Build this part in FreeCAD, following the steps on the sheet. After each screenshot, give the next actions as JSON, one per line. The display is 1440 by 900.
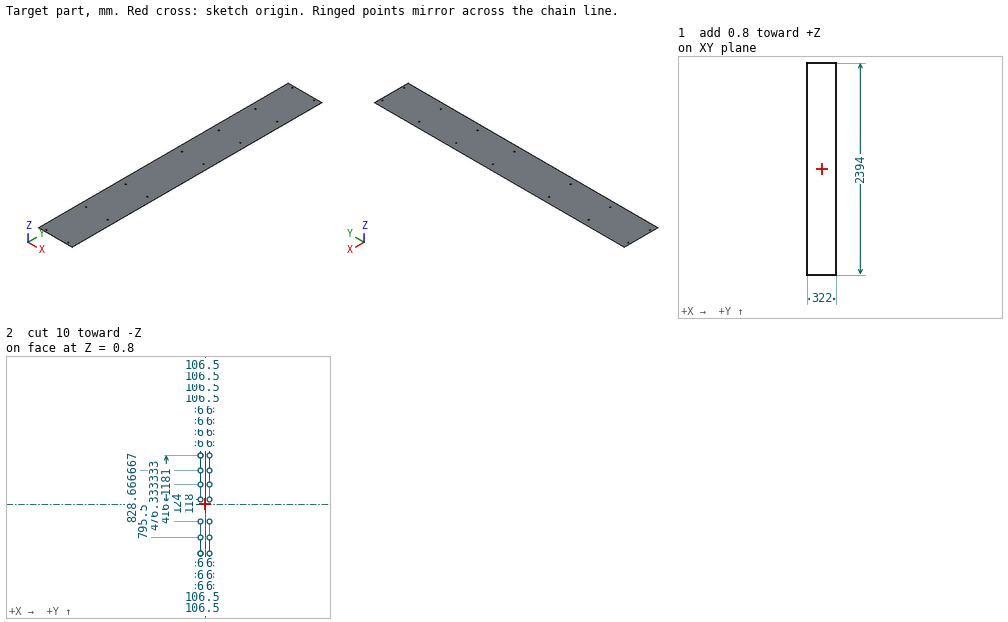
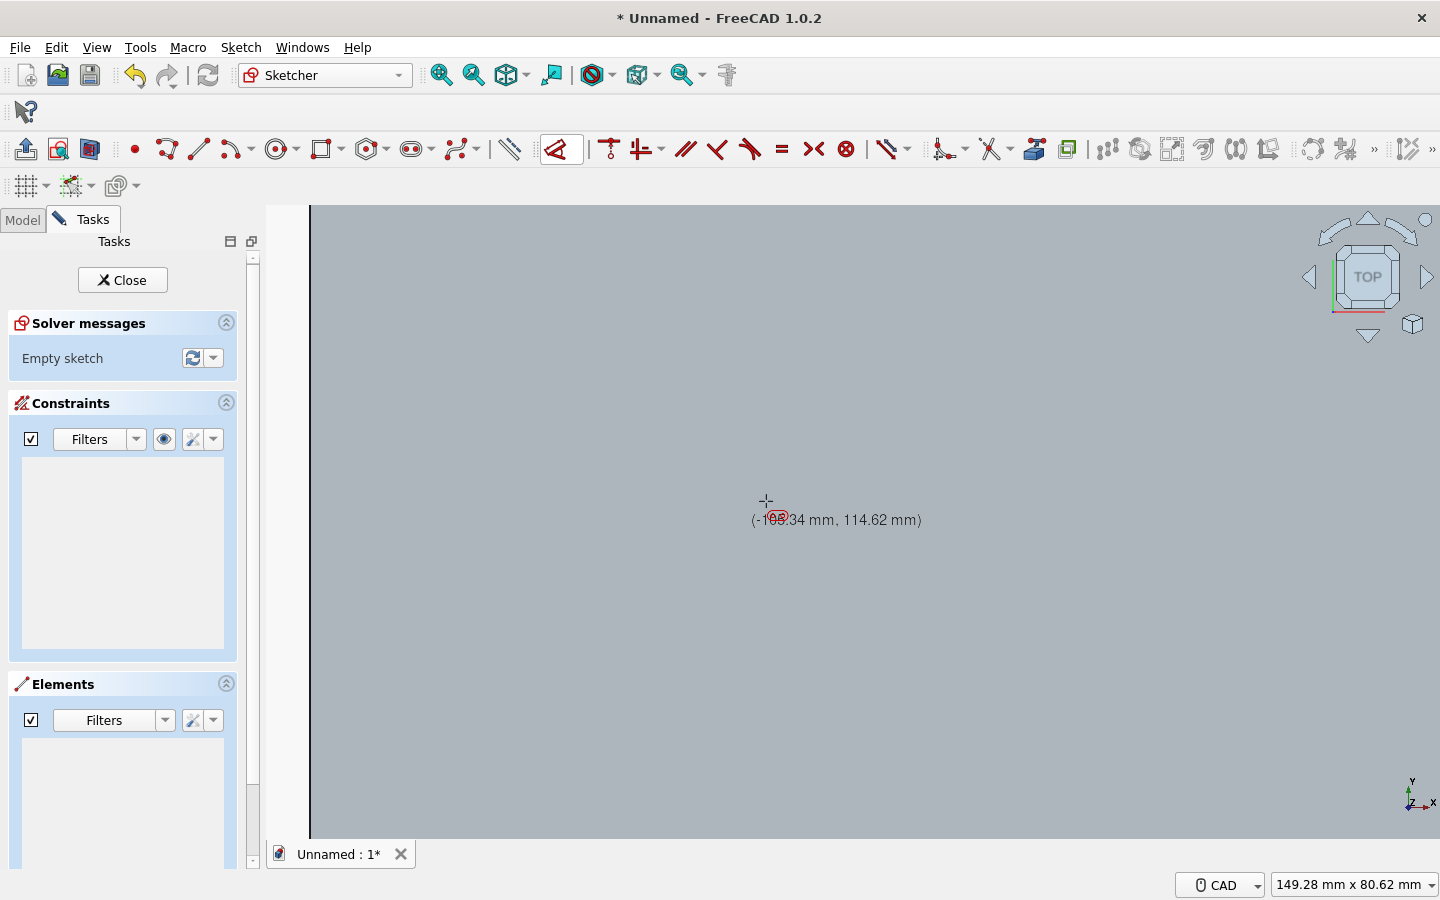
{"action": "scroll", "coordinate": [762, 497], "scroll_direction": "down", "scroll_amount": 18}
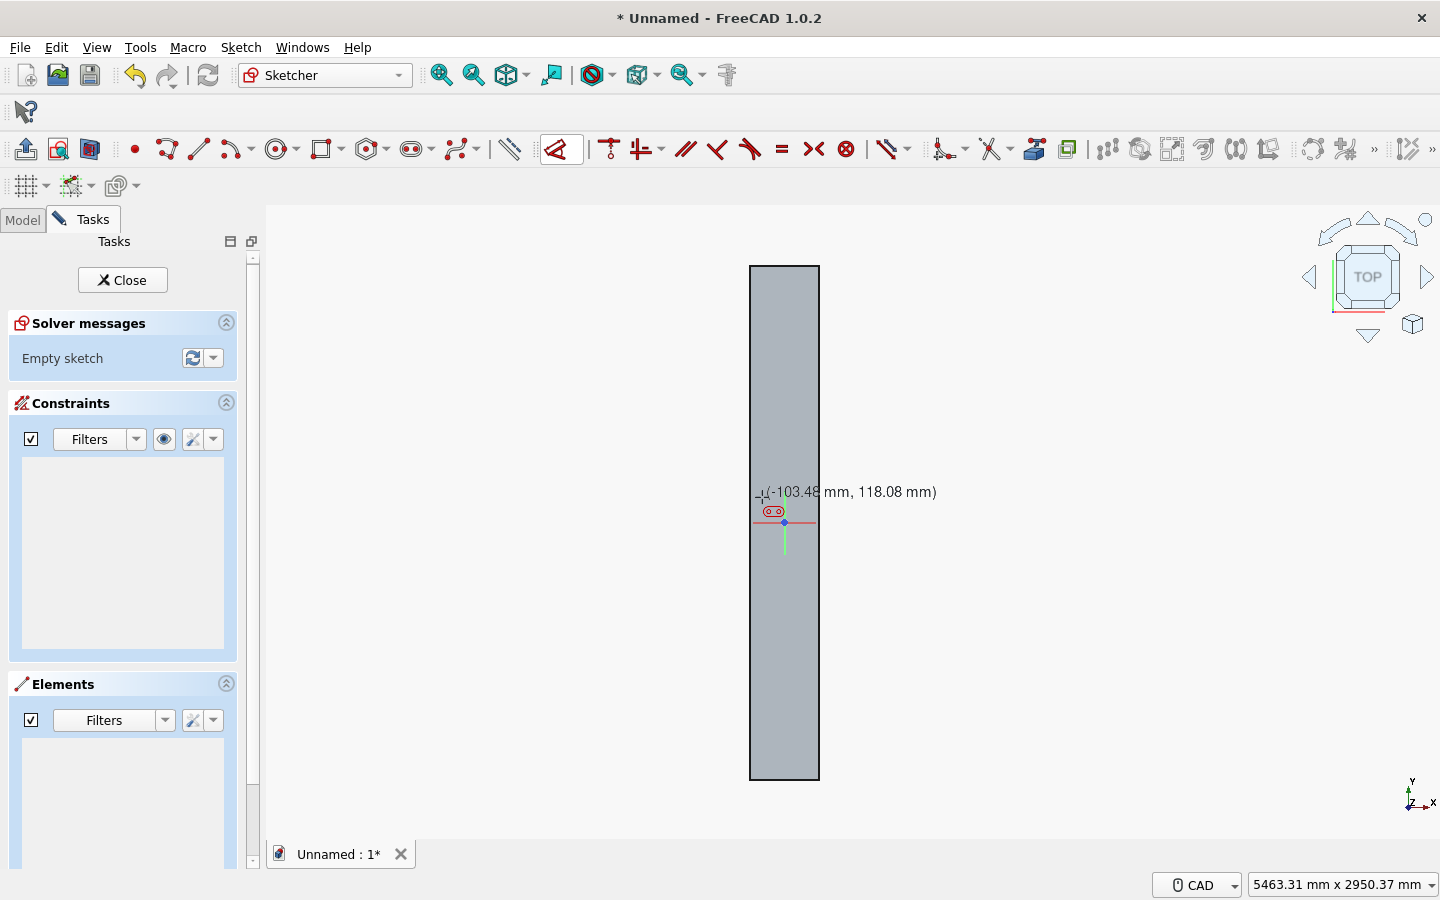
{"action": "left_click", "coordinate": [762, 497]}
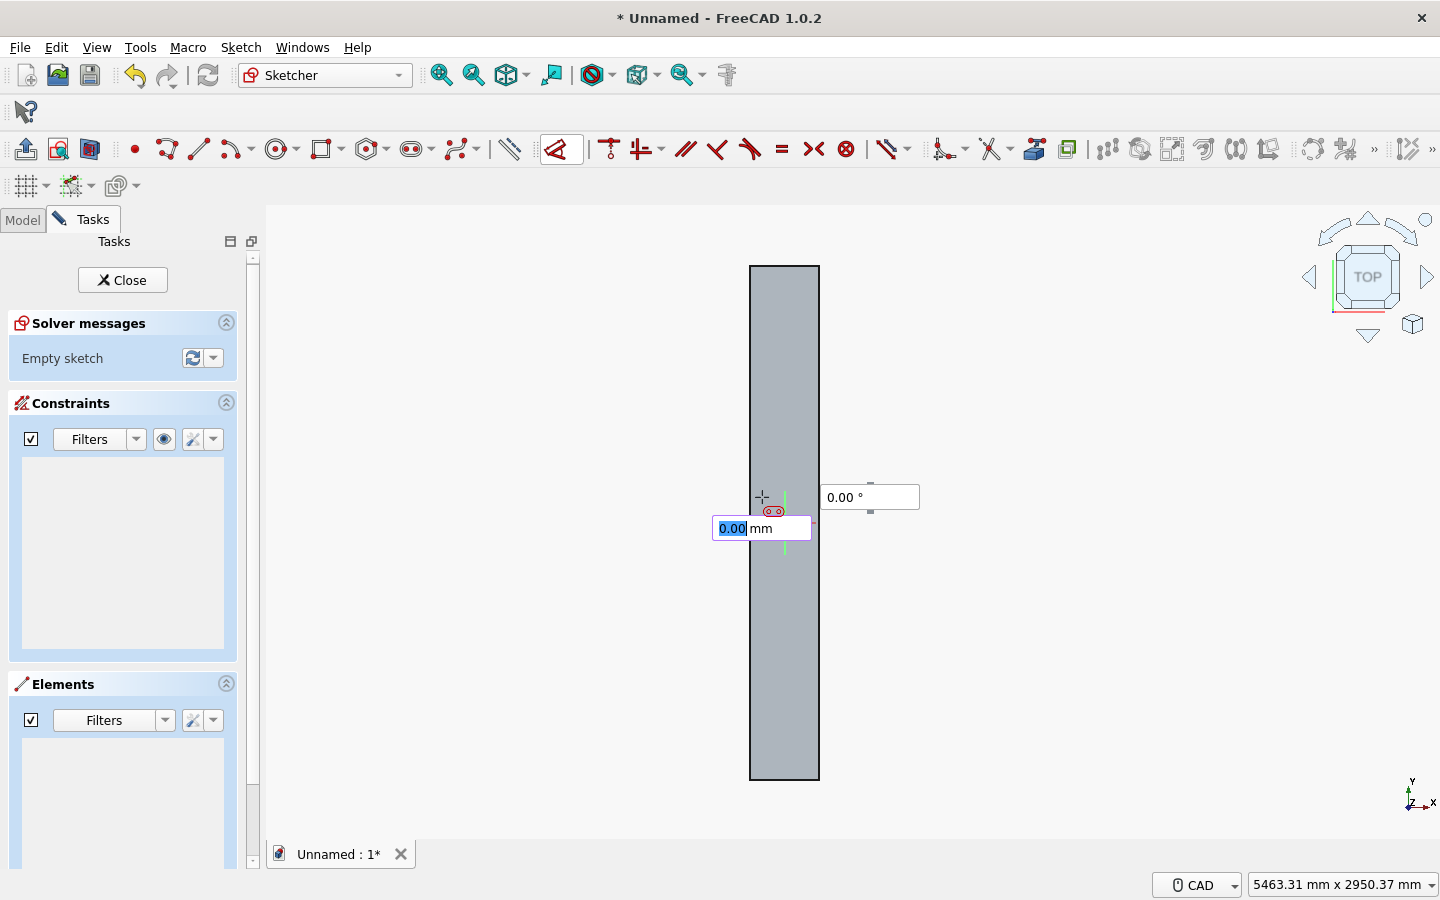
{"action": "scroll", "coordinate": [763, 497], "scroll_direction": "up", "scroll_amount": 13}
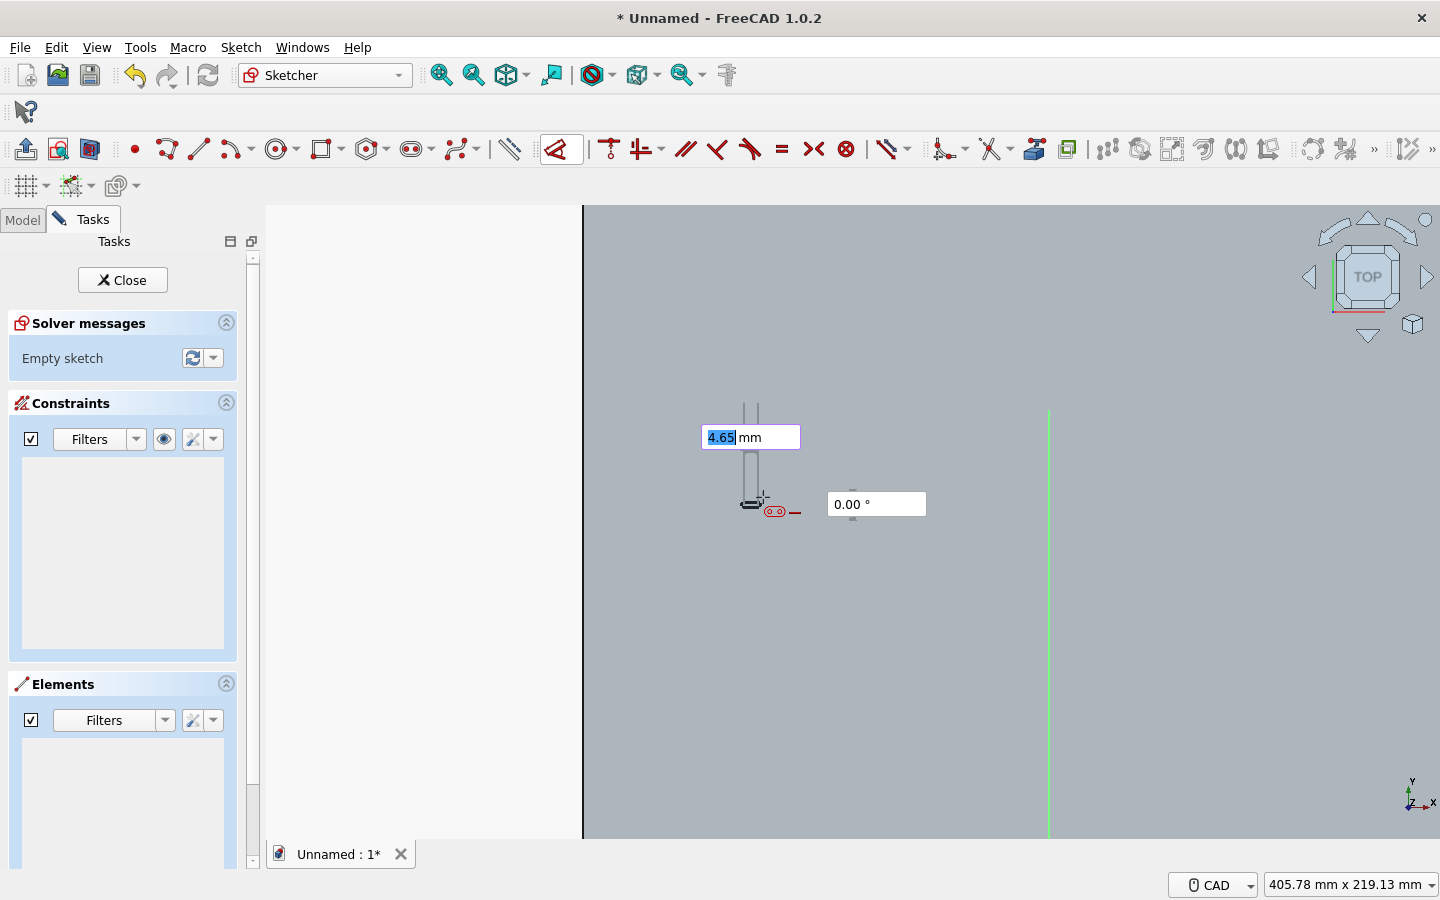
{"action": "left_click", "coordinate": [758, 491]}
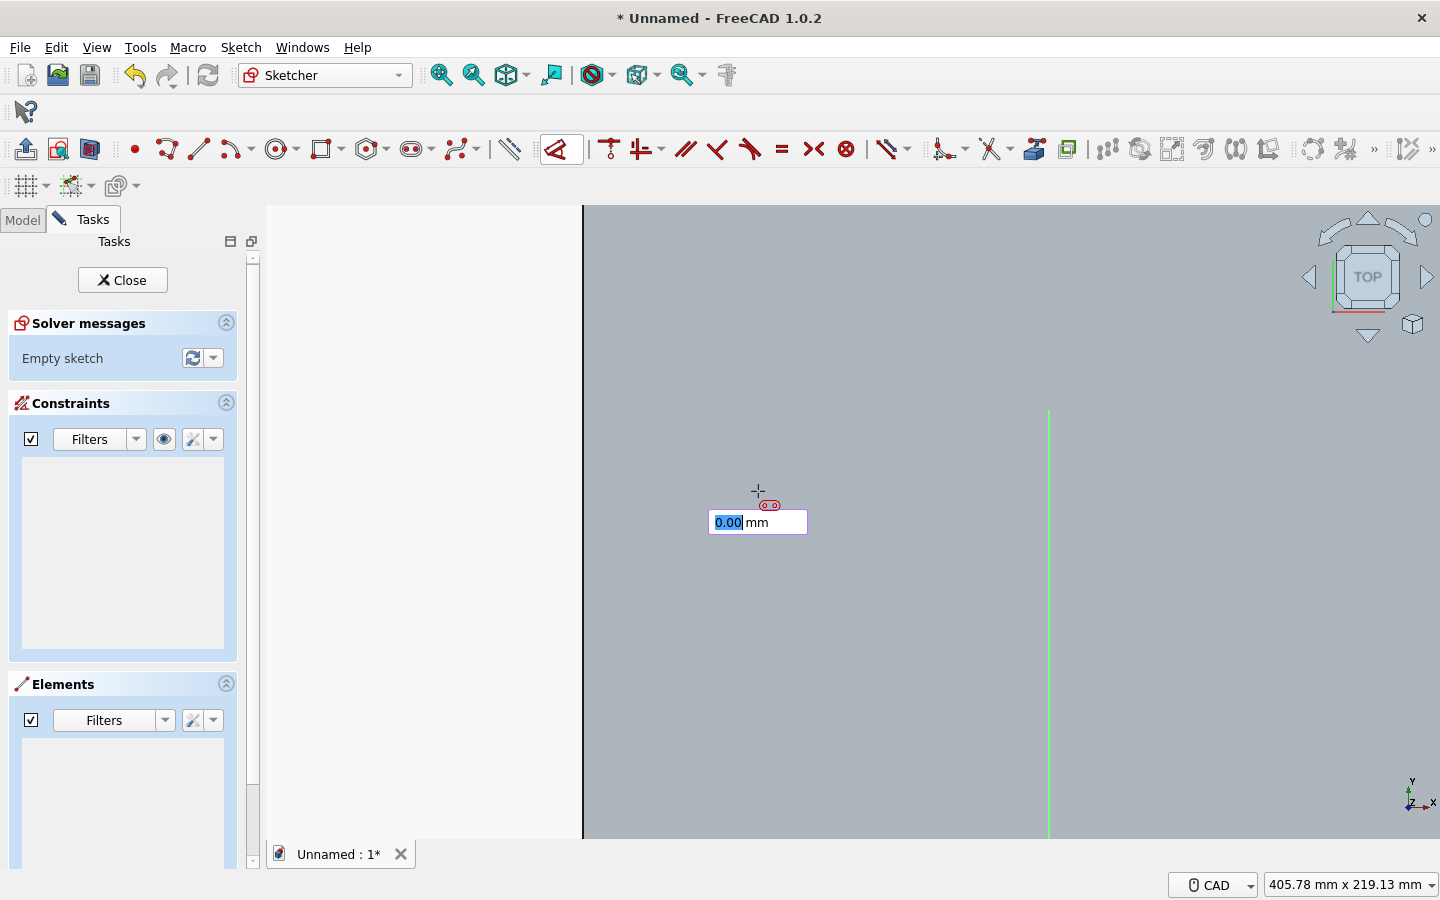
{"action": "scroll", "coordinate": [750, 481], "scroll_direction": "up", "scroll_amount": 4}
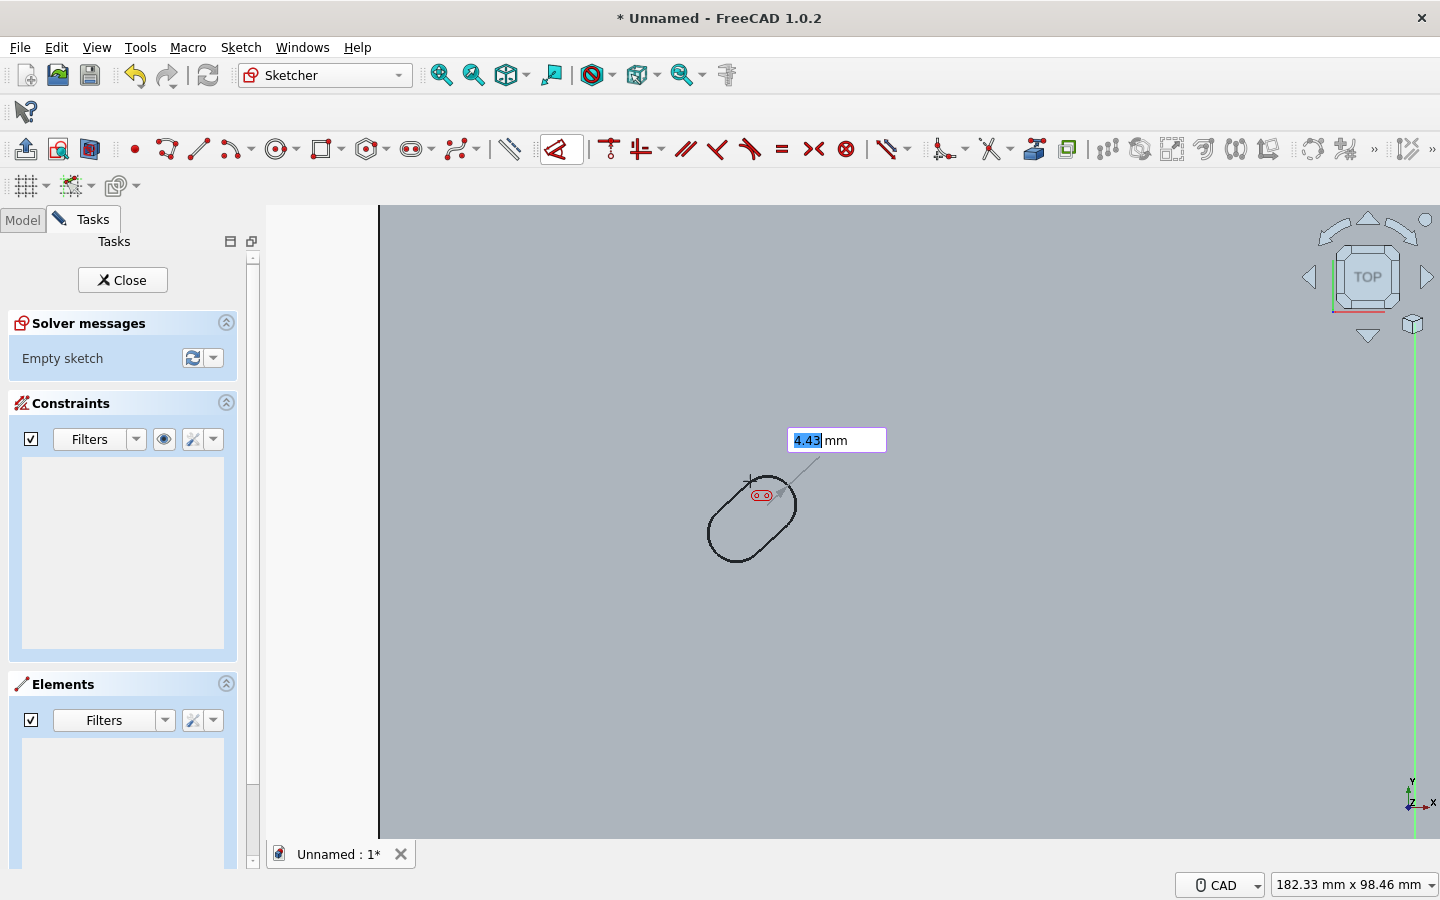
{"action": "left_click", "coordinate": [749, 479]}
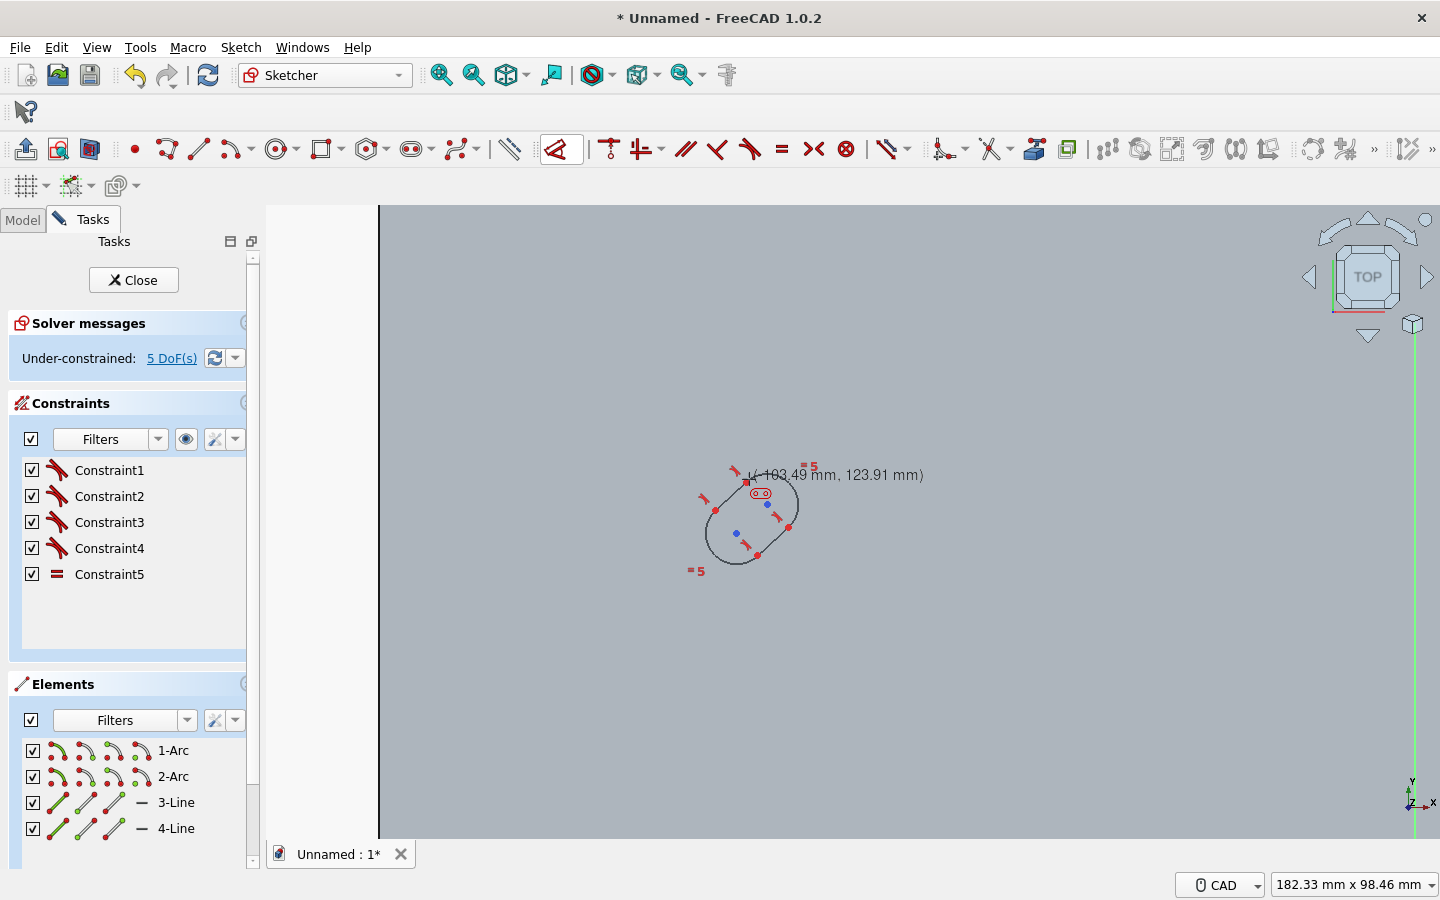
{"action": "scroll", "coordinate": [763, 496], "scroll_direction": "down", "scroll_amount": 17}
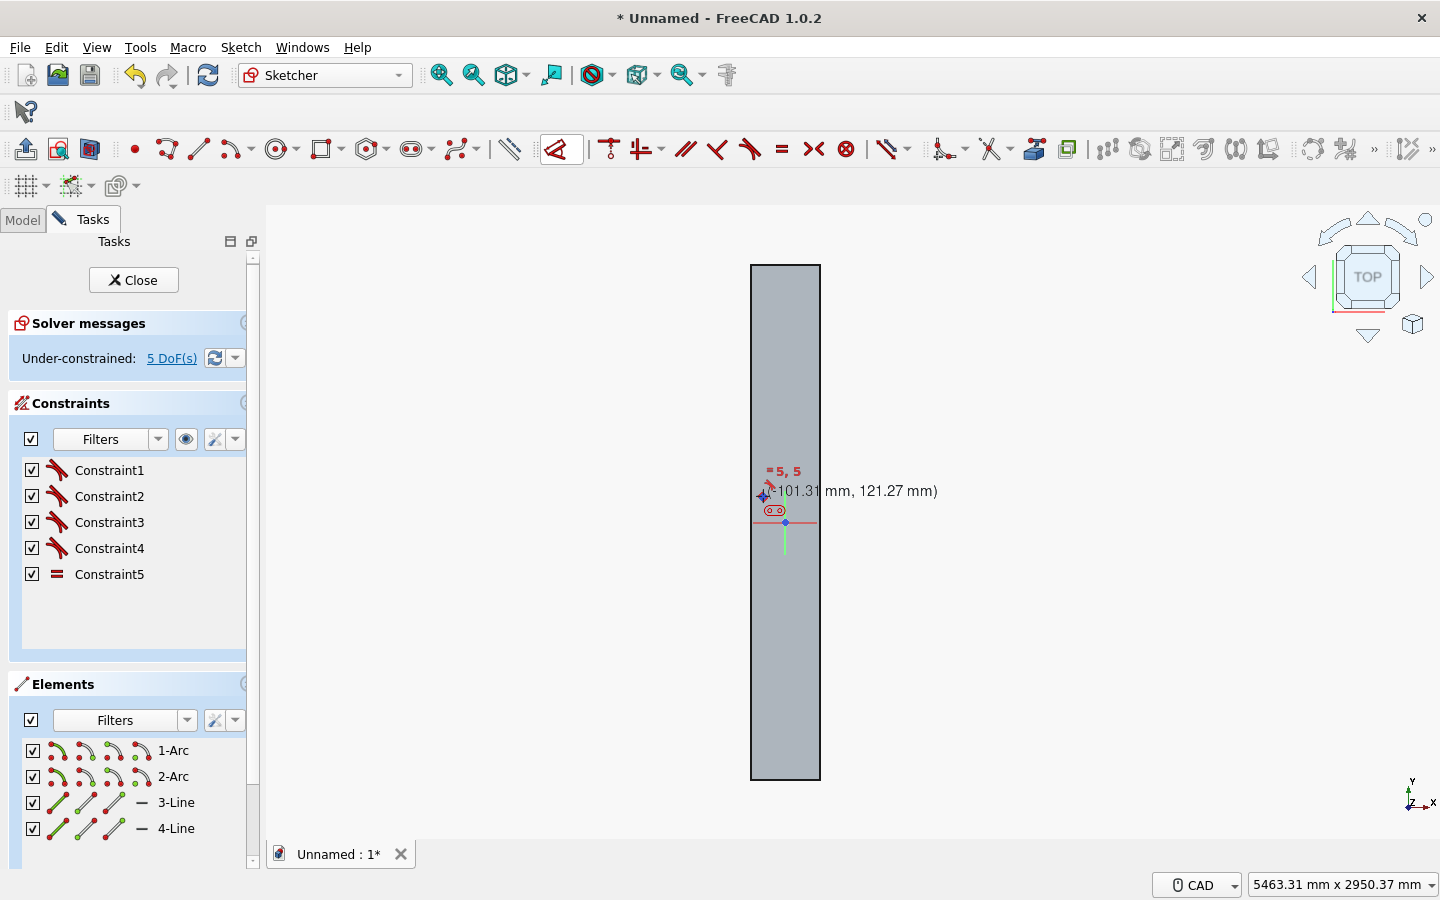
{"action": "scroll", "coordinate": [762, 269], "scroll_direction": "up", "scroll_amount": 18}